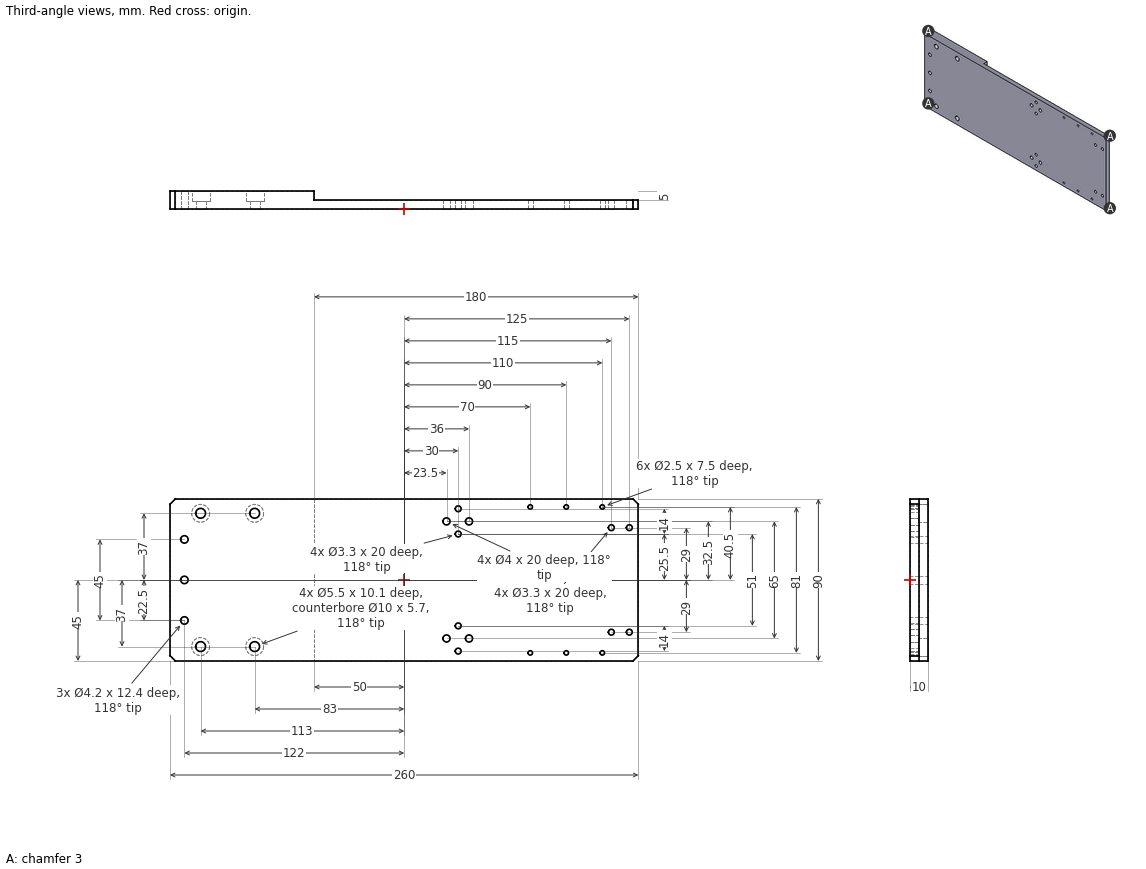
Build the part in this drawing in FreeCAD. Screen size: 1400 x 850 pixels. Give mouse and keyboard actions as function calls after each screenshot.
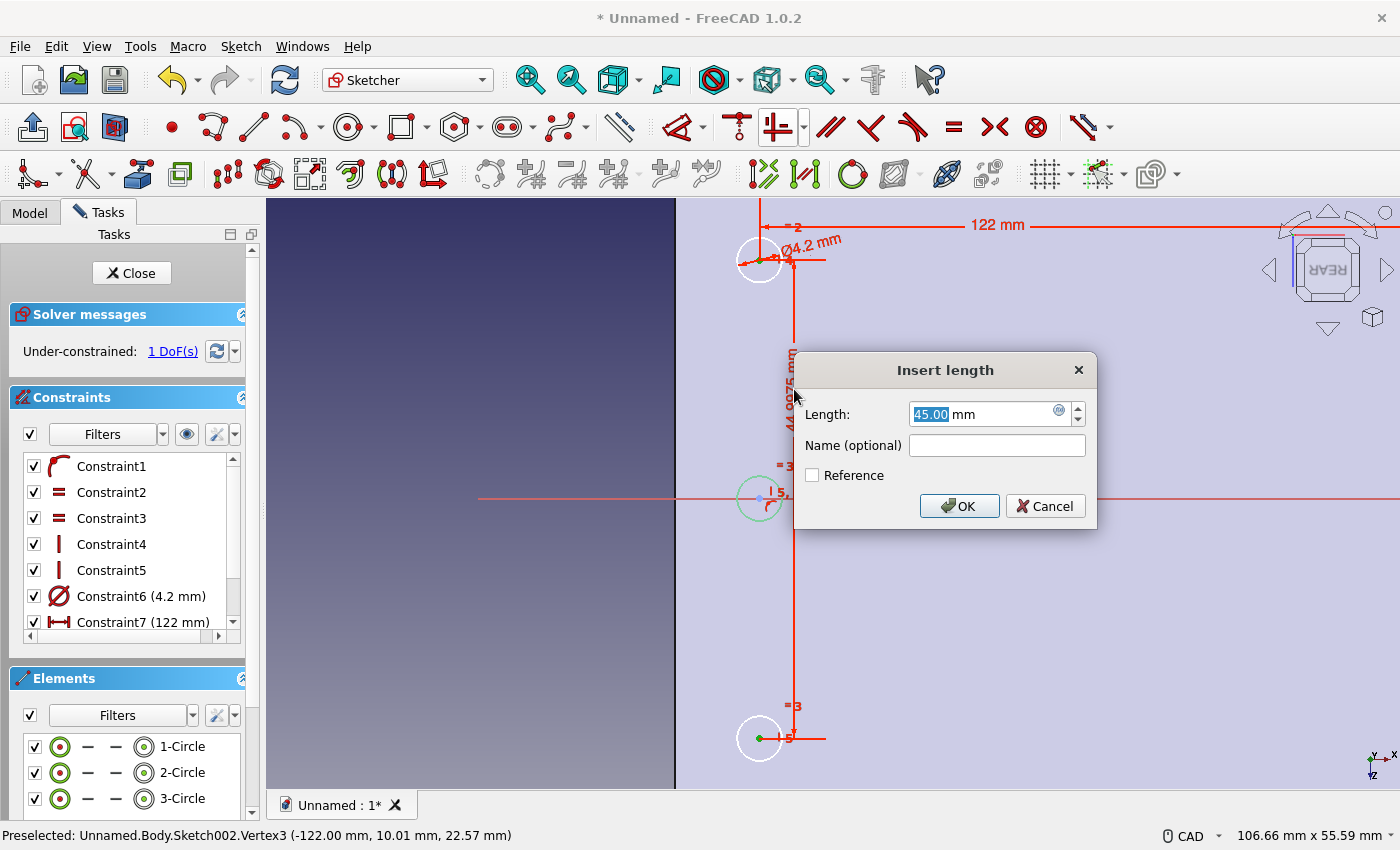
text(45)
key(Return)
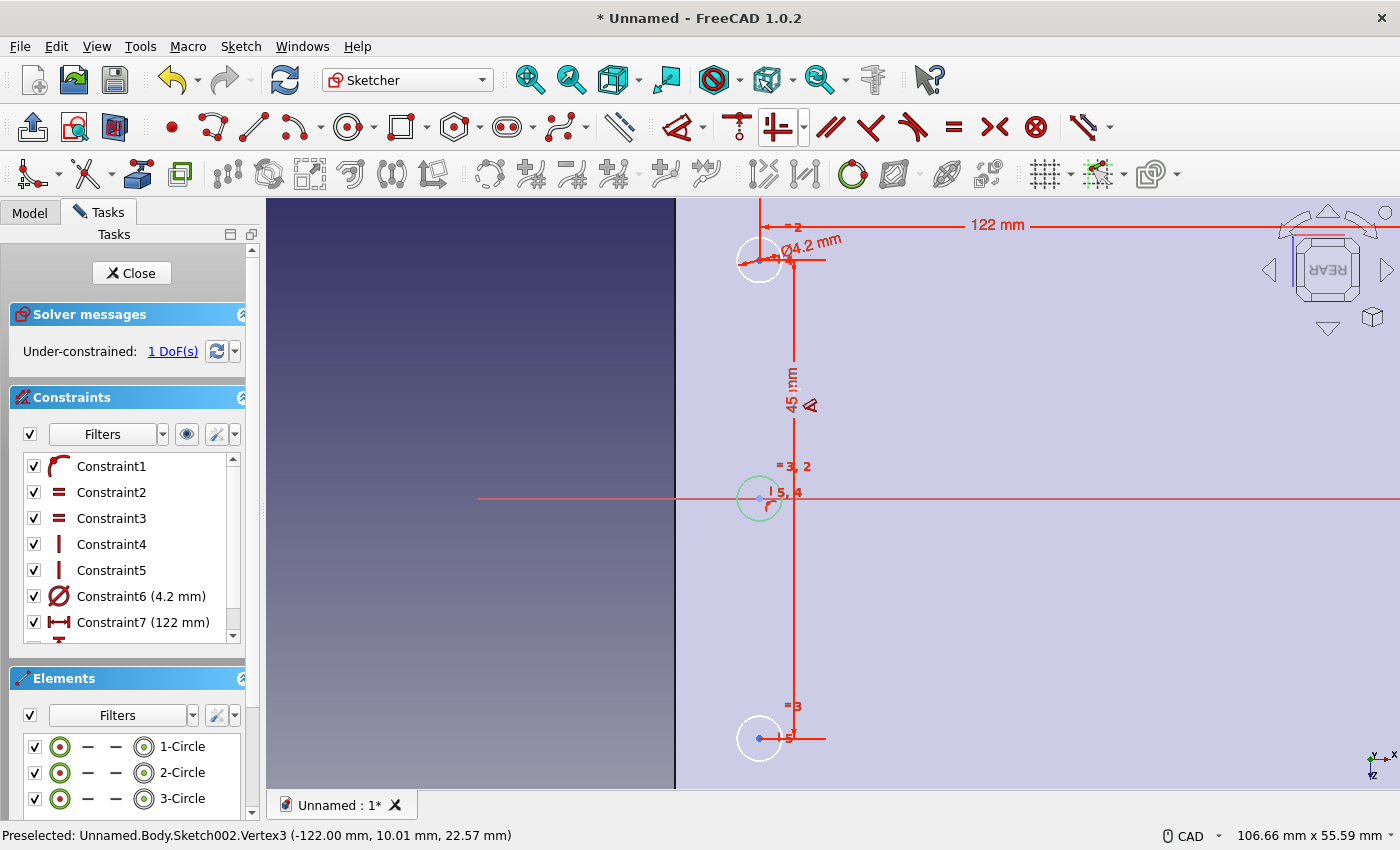
click(760, 260)
click(726, 325)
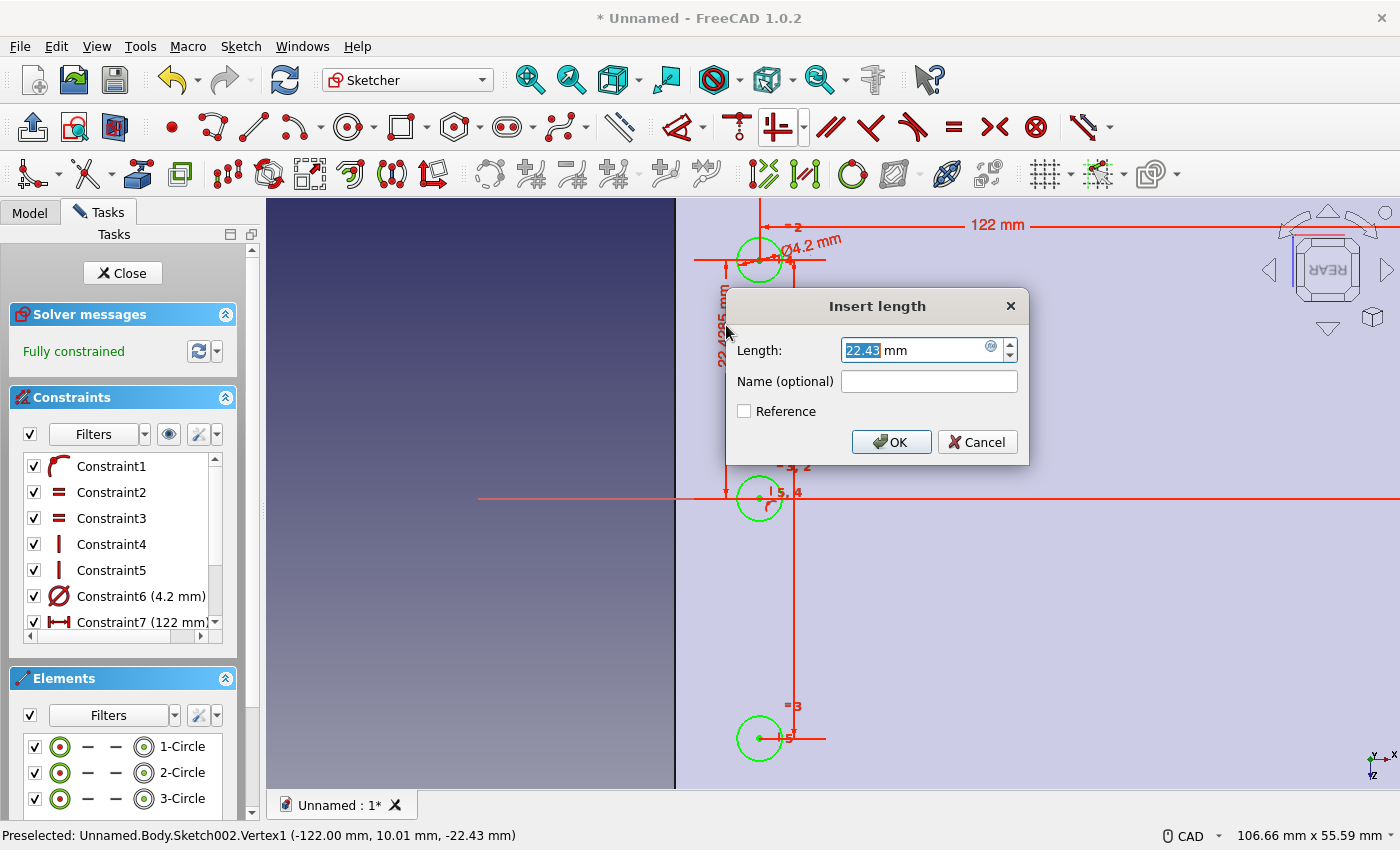
text(22.5)
key(Return)
key(Escape)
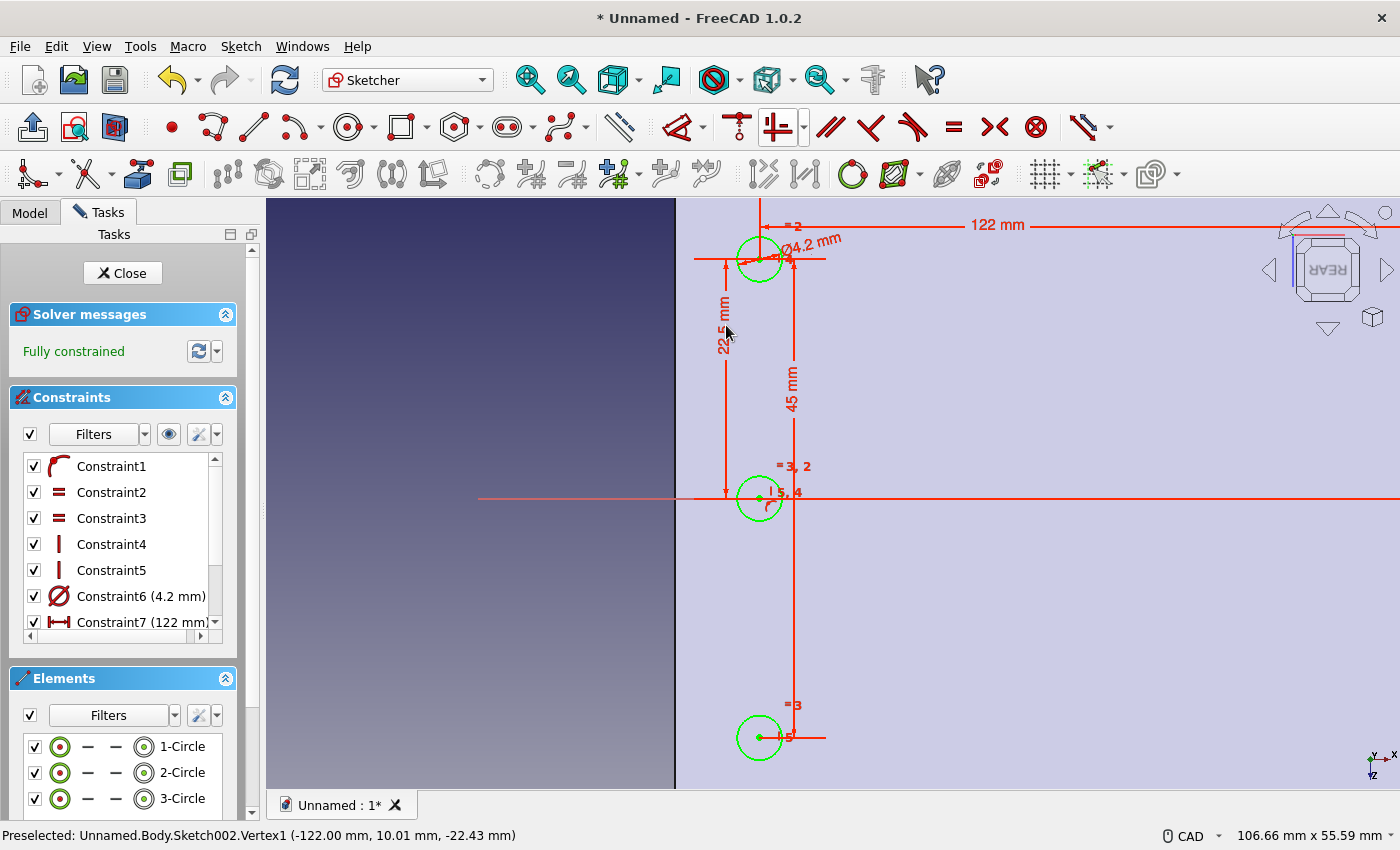
click(123, 273)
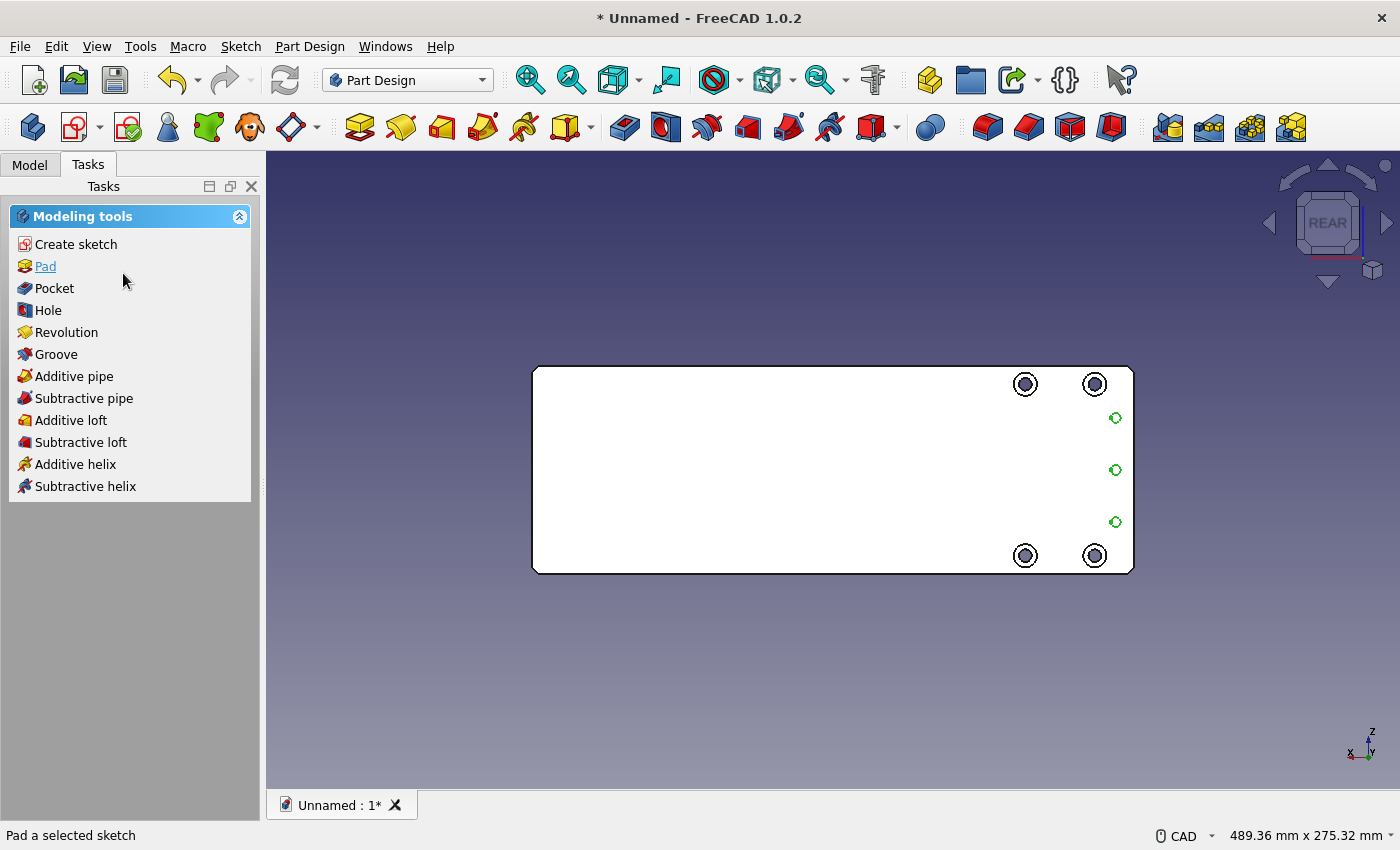
click(666, 128)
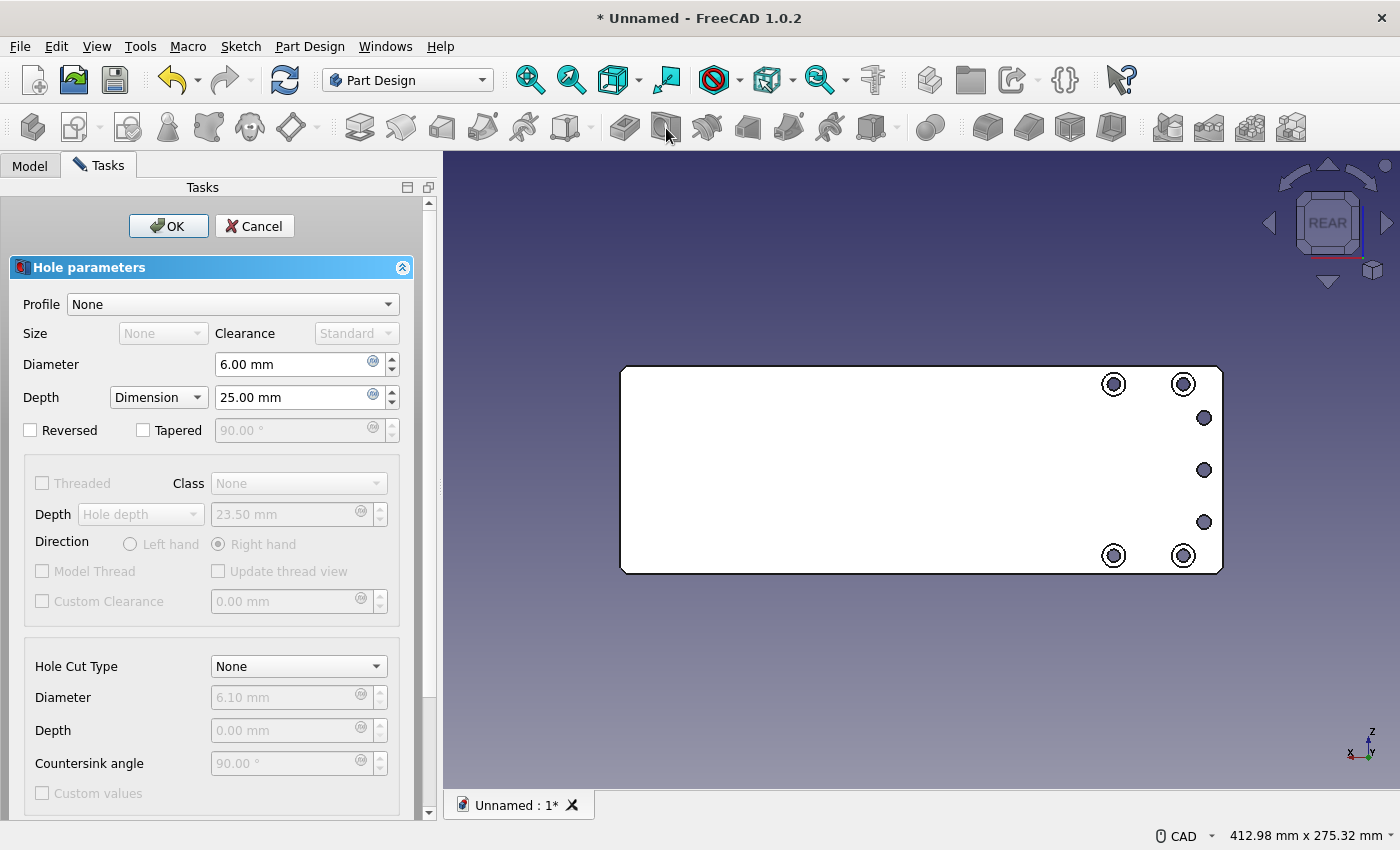
triple_click(300, 364)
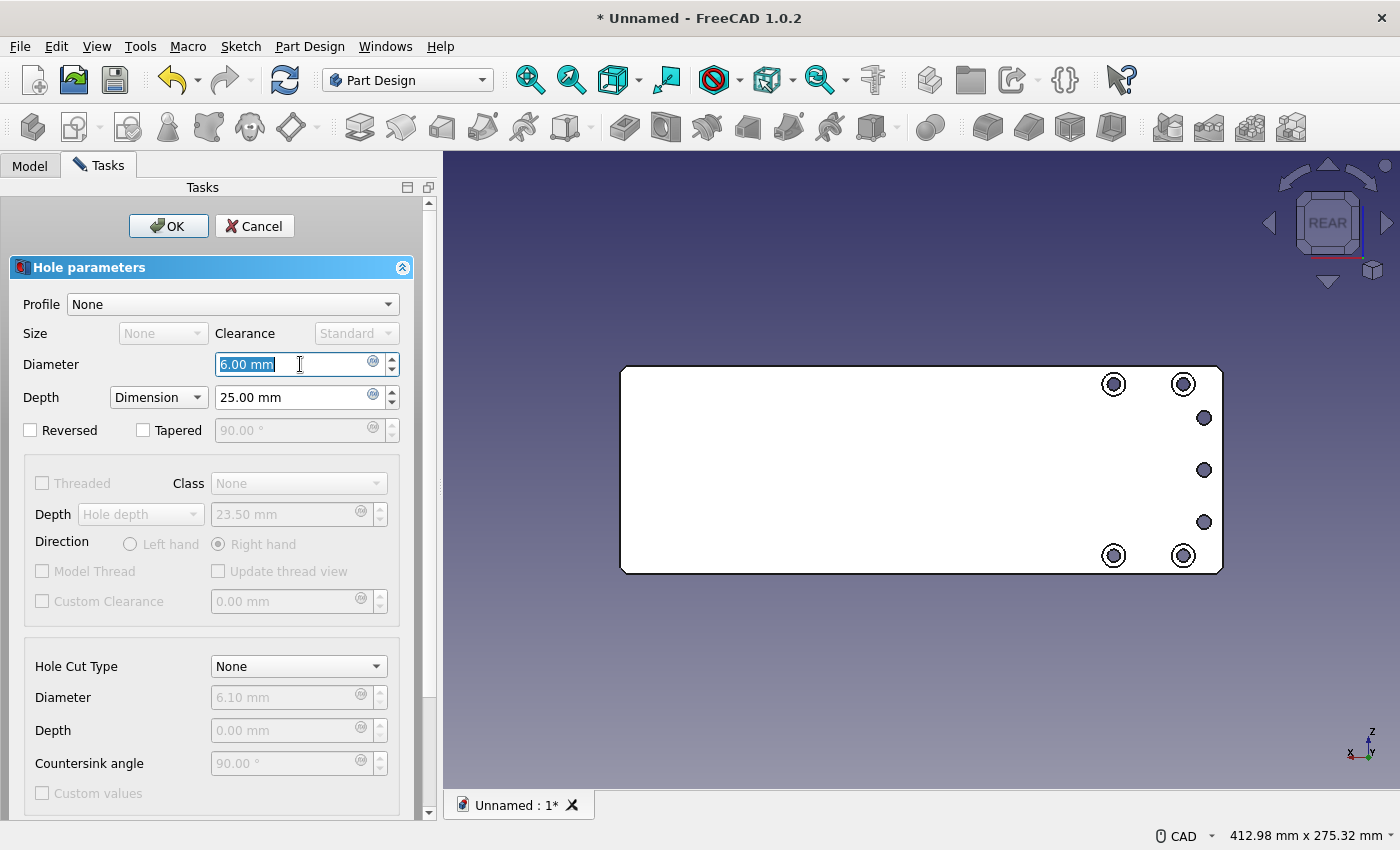
text(4.2)
key(Tab)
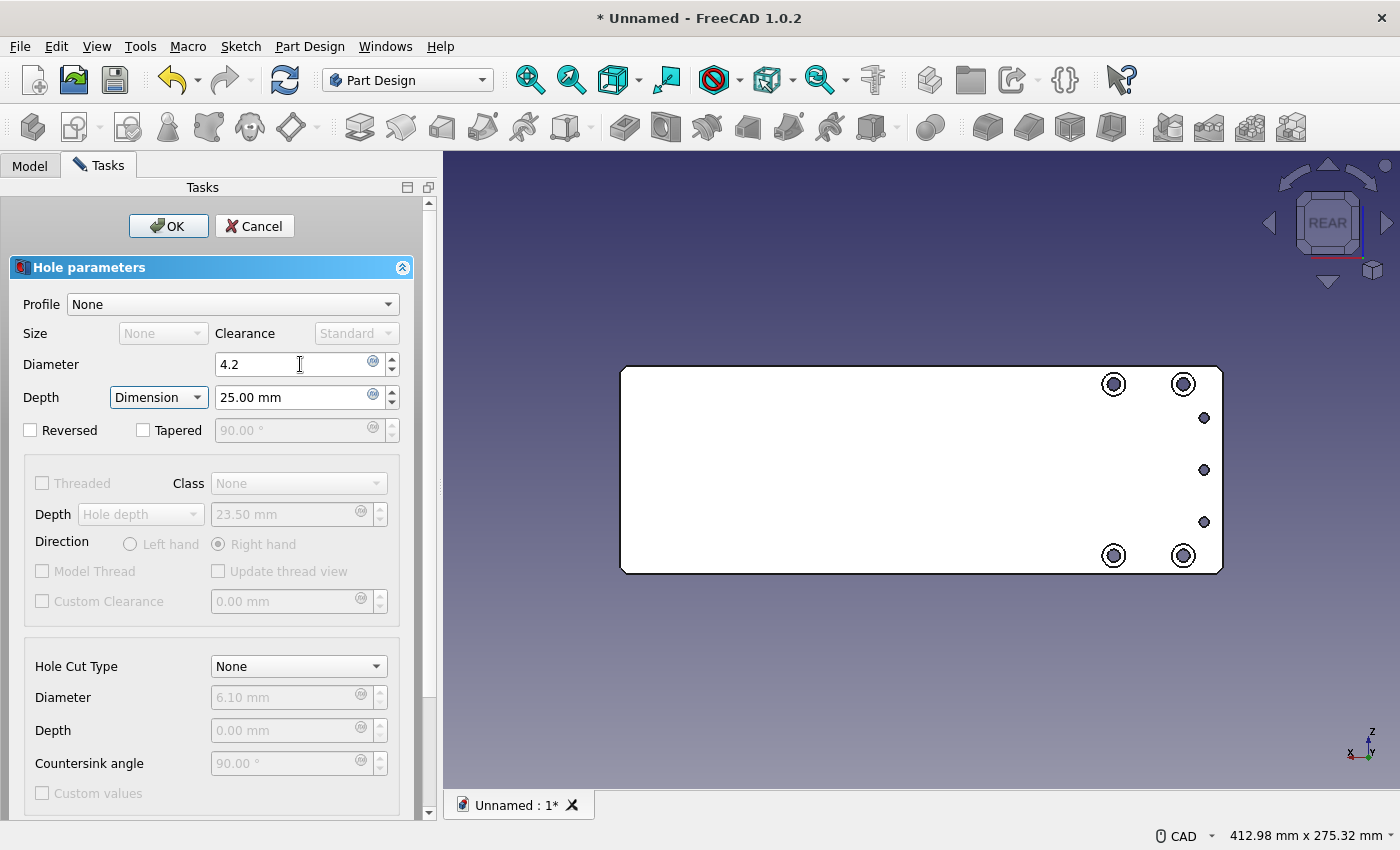
triple_click(300, 398)